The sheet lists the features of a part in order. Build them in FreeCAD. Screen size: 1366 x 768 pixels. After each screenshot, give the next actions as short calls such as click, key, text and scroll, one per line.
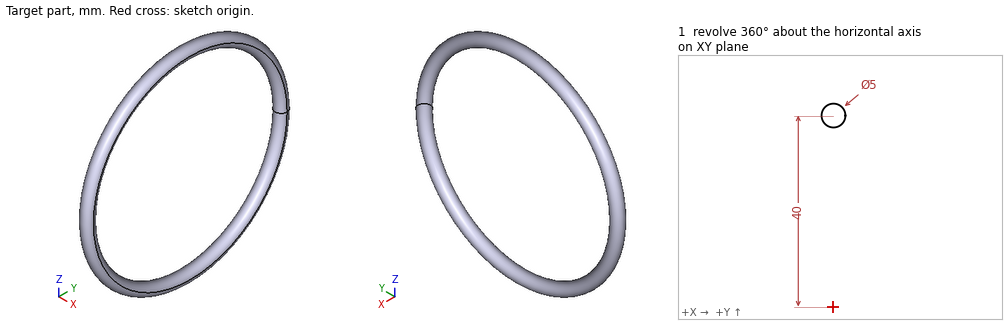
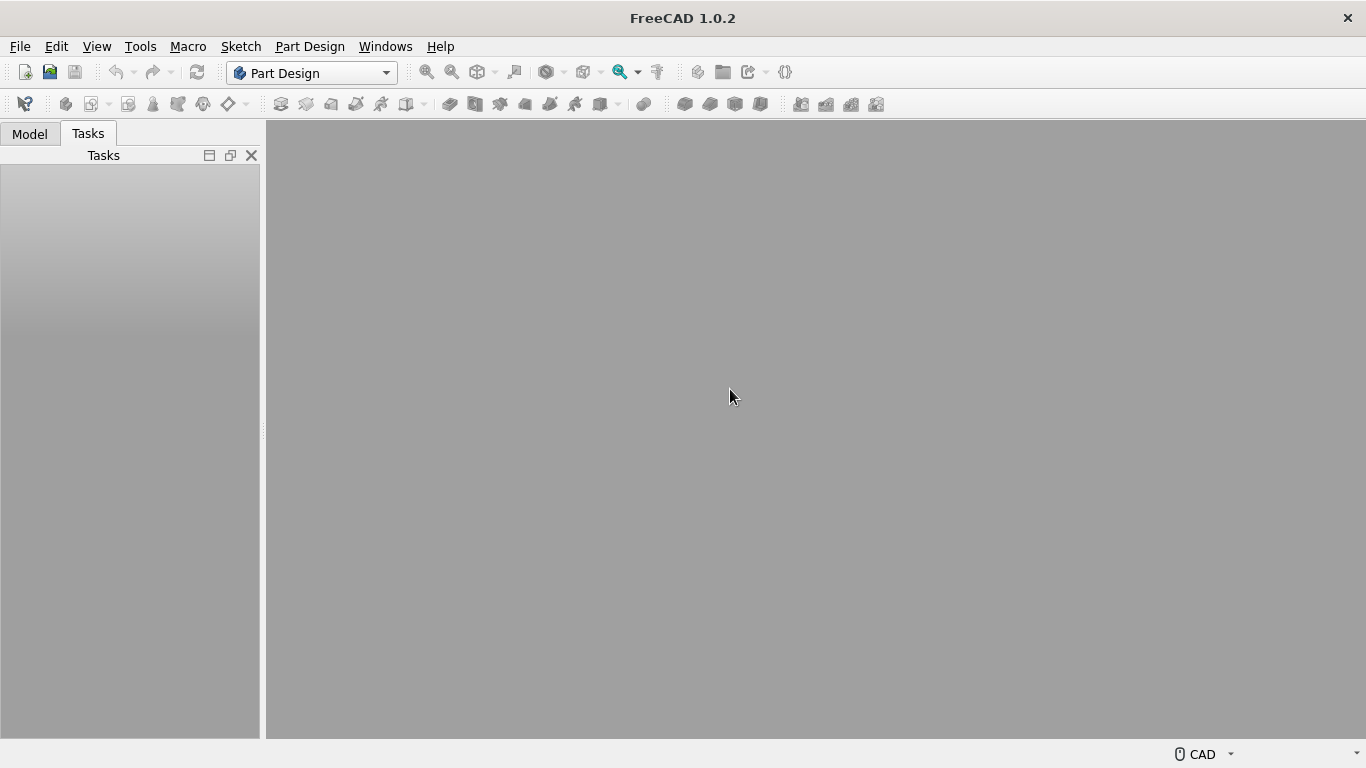
click(25, 72)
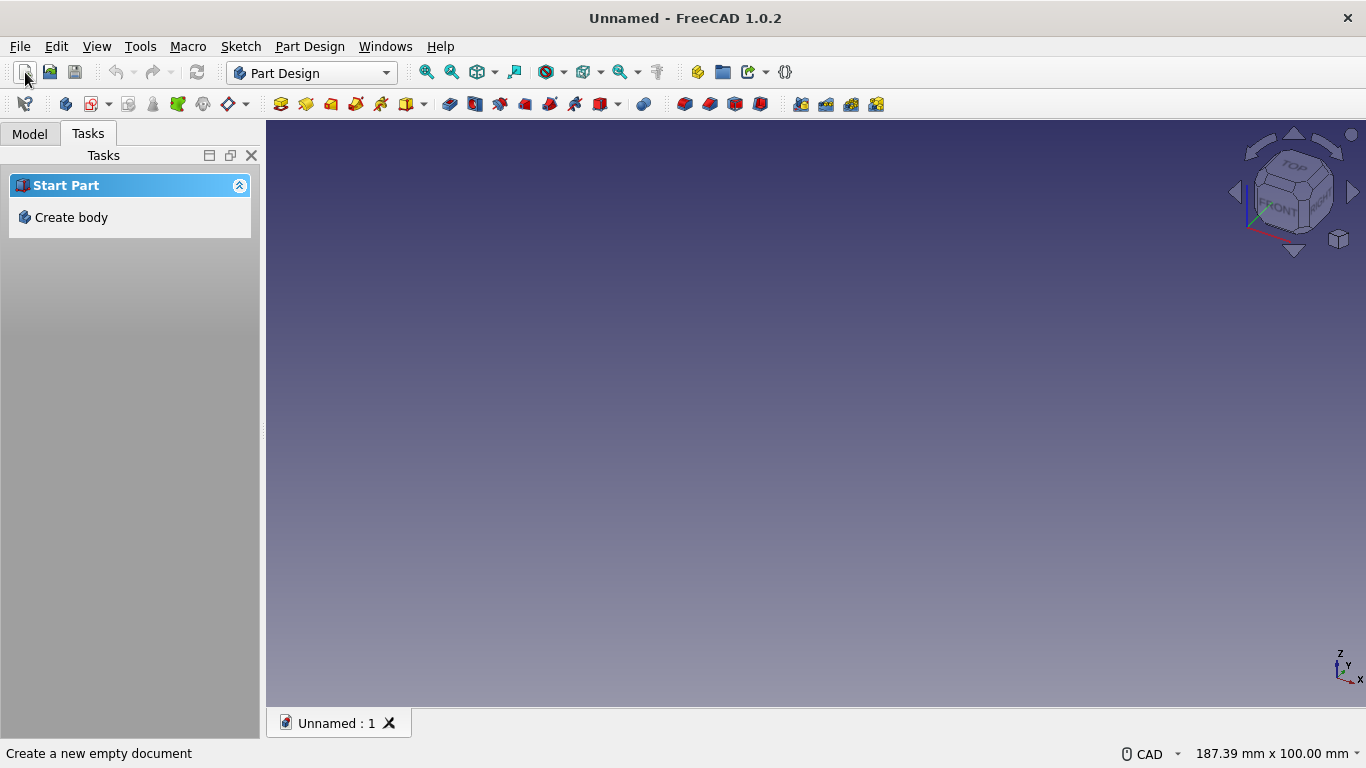
click(90, 104)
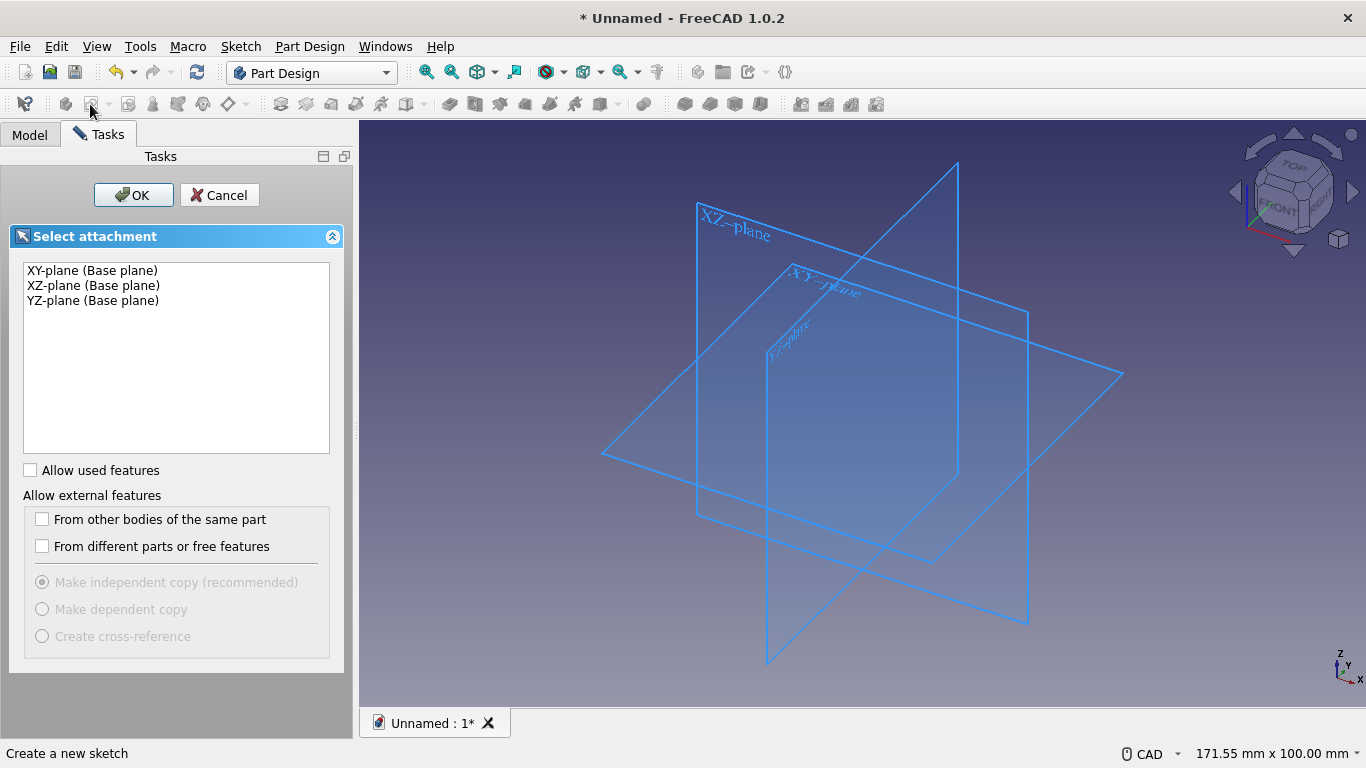
click(84, 270)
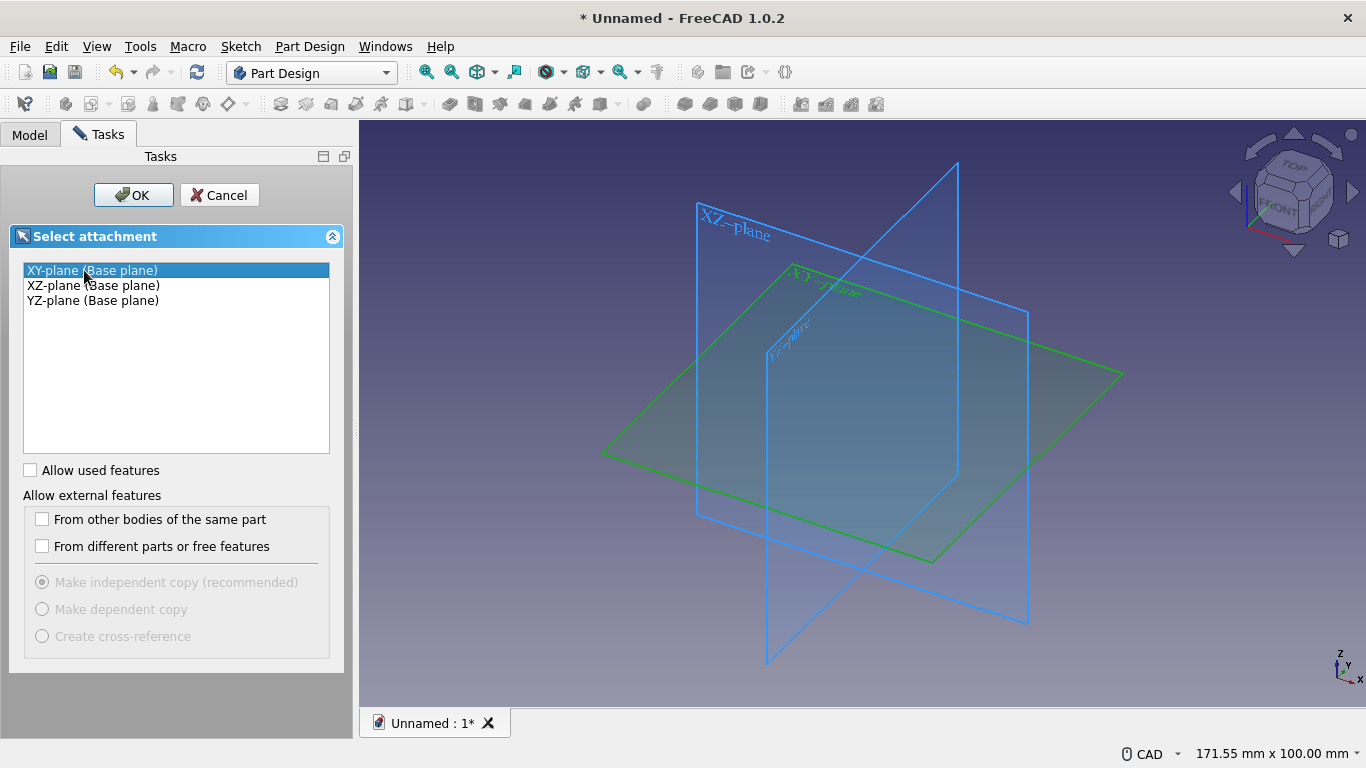
click(134, 195)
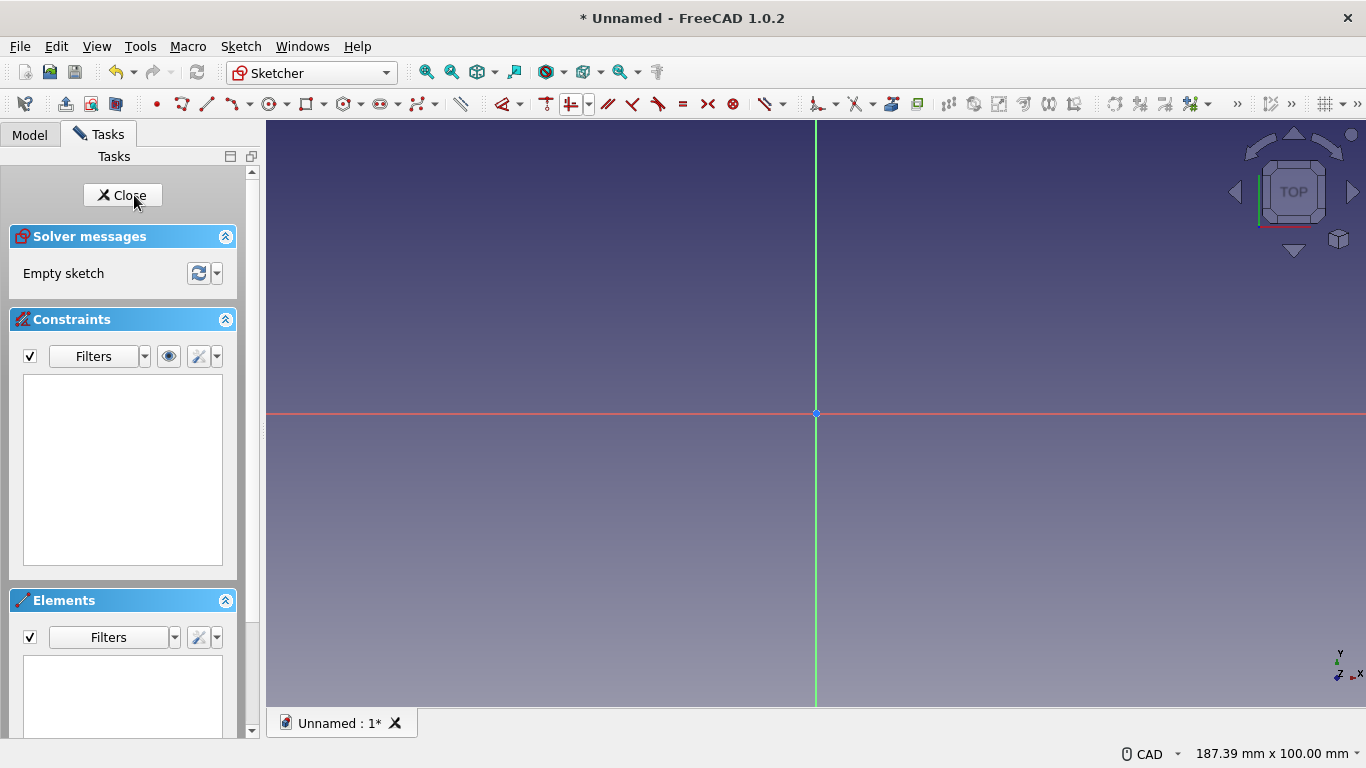
scroll(821, 160, up, 13)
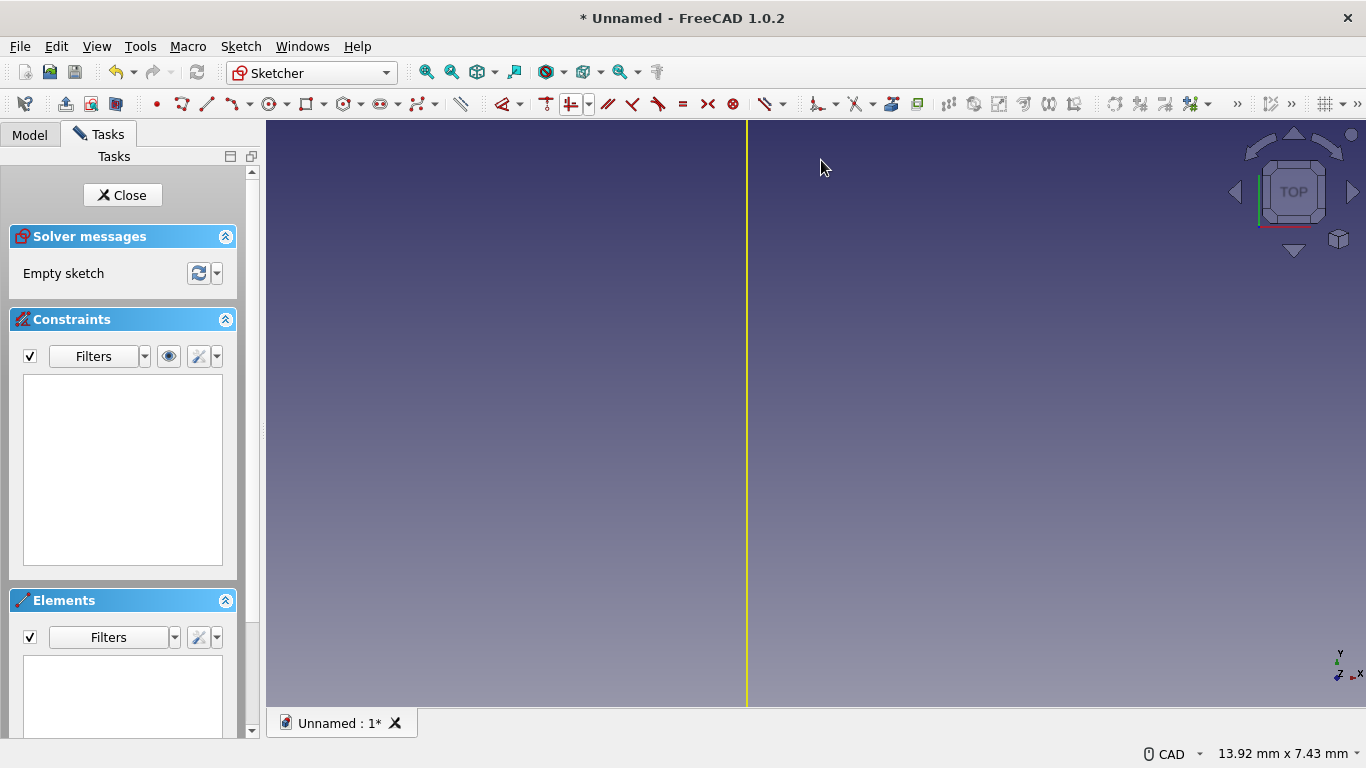
click(268, 104)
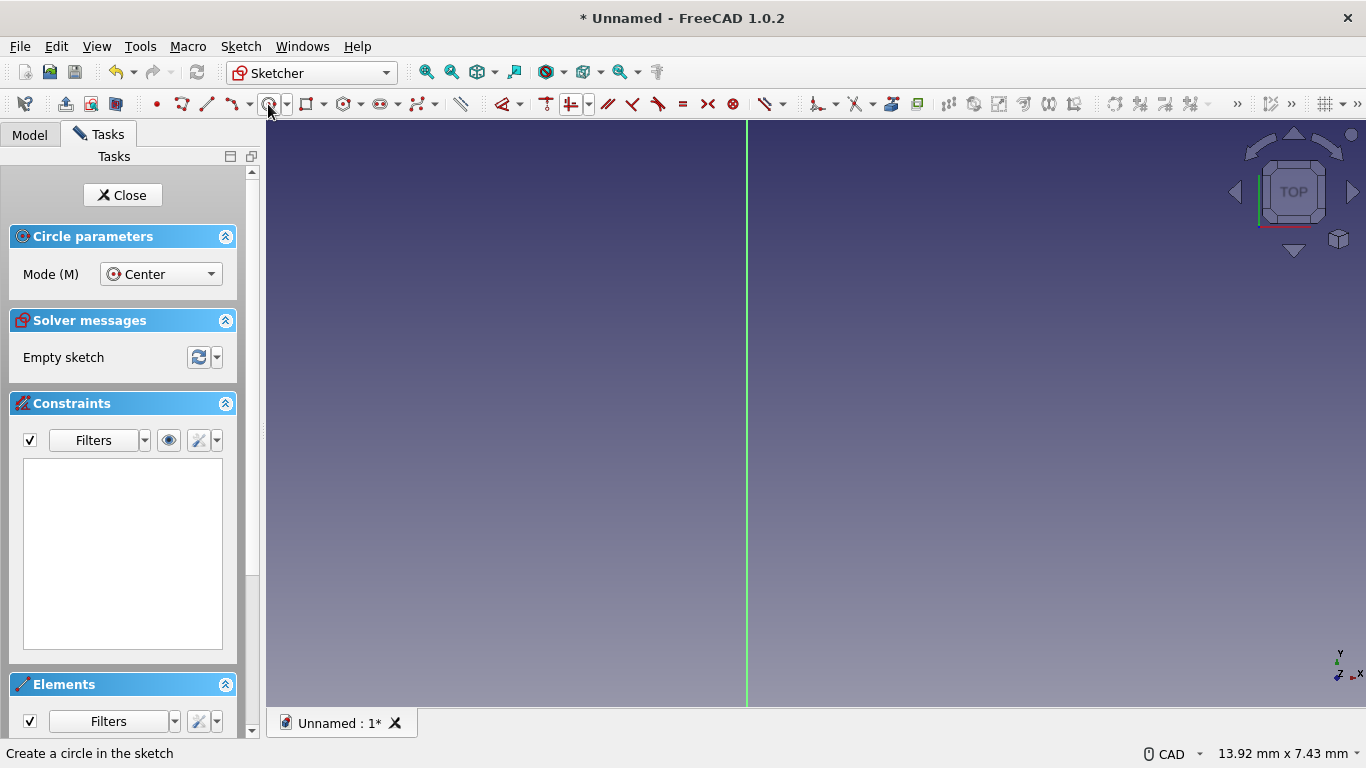
click(747, 411)
click(887, 271)
key(Escape)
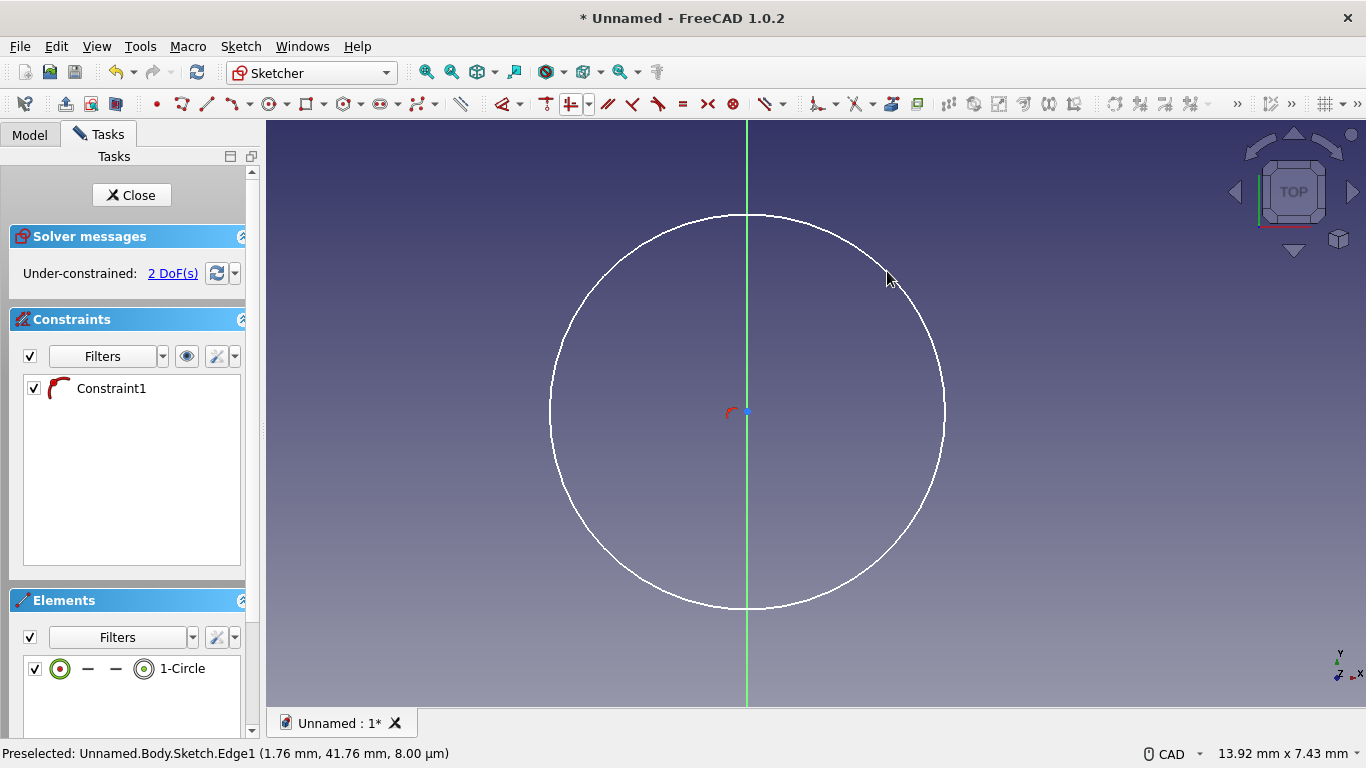
click(887, 272)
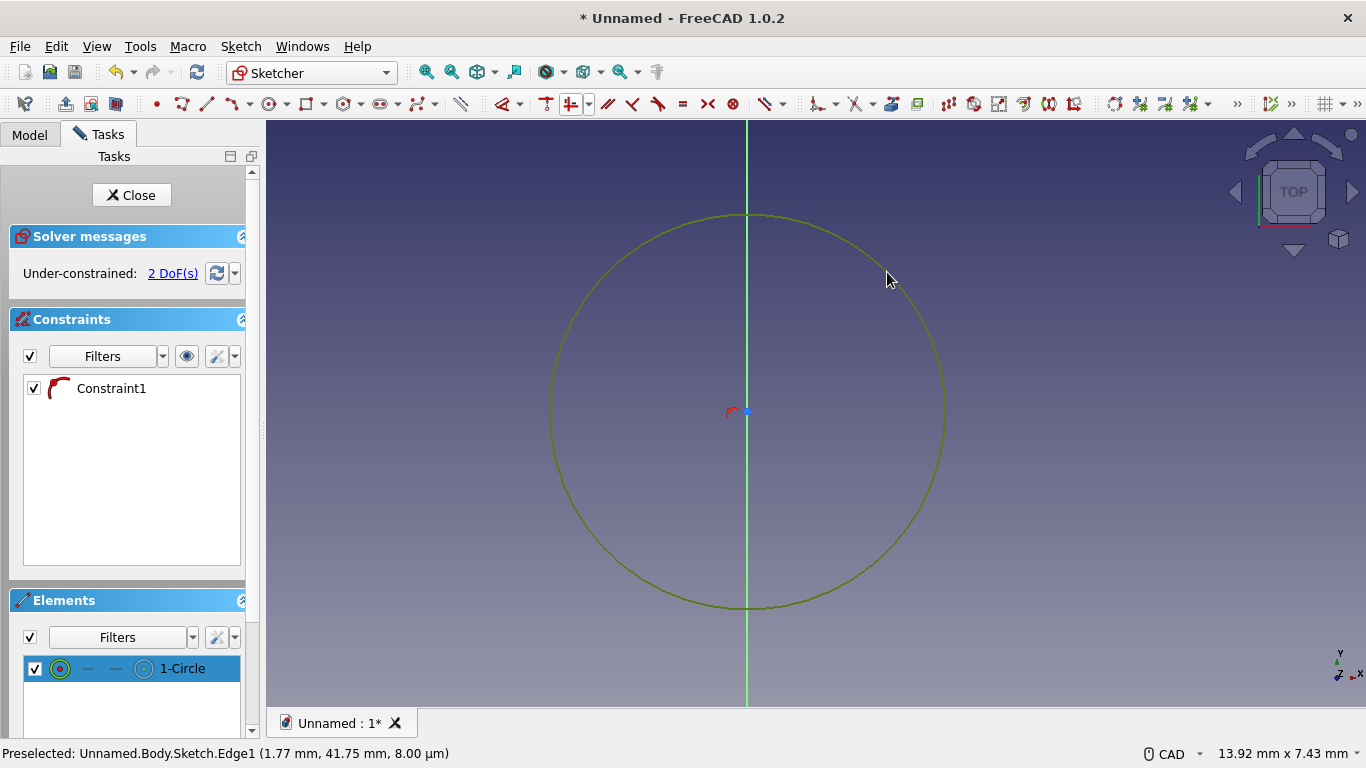
click(520, 104)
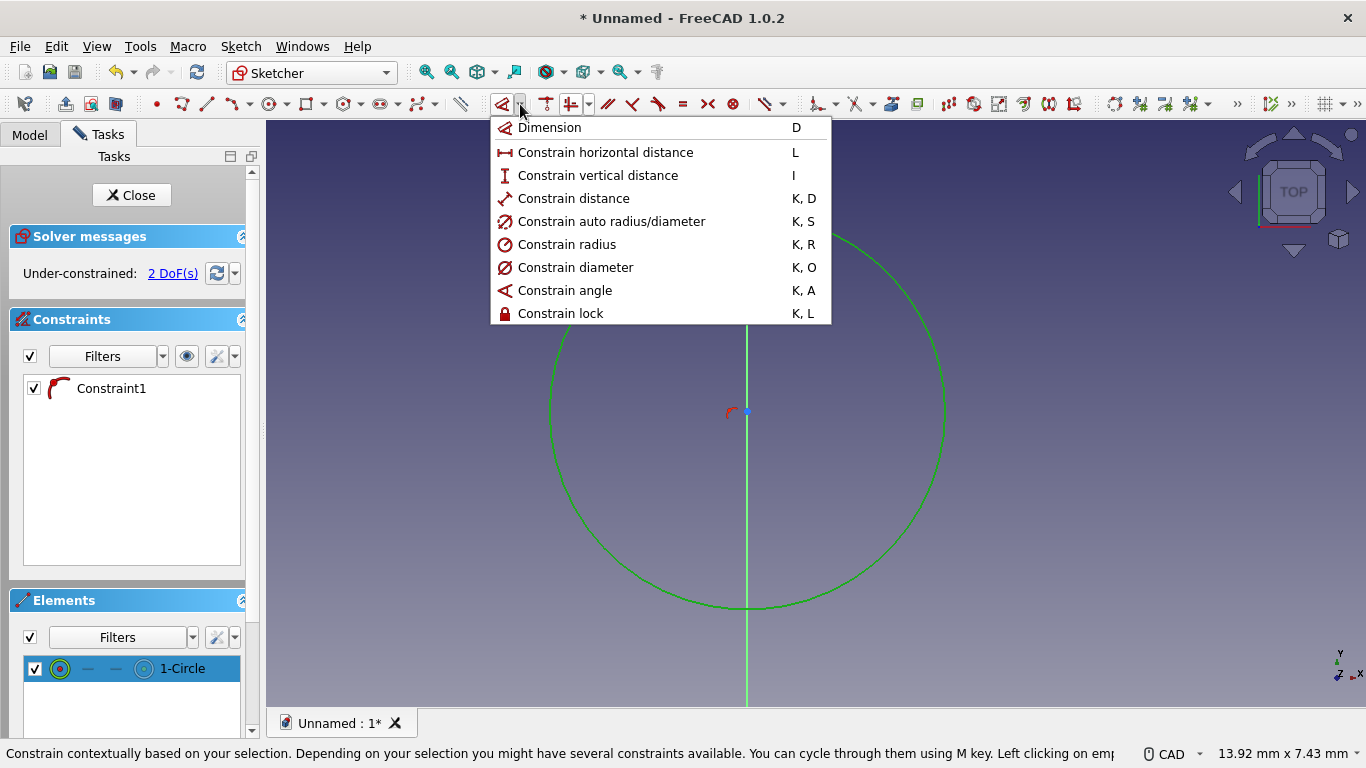
click(661, 268)